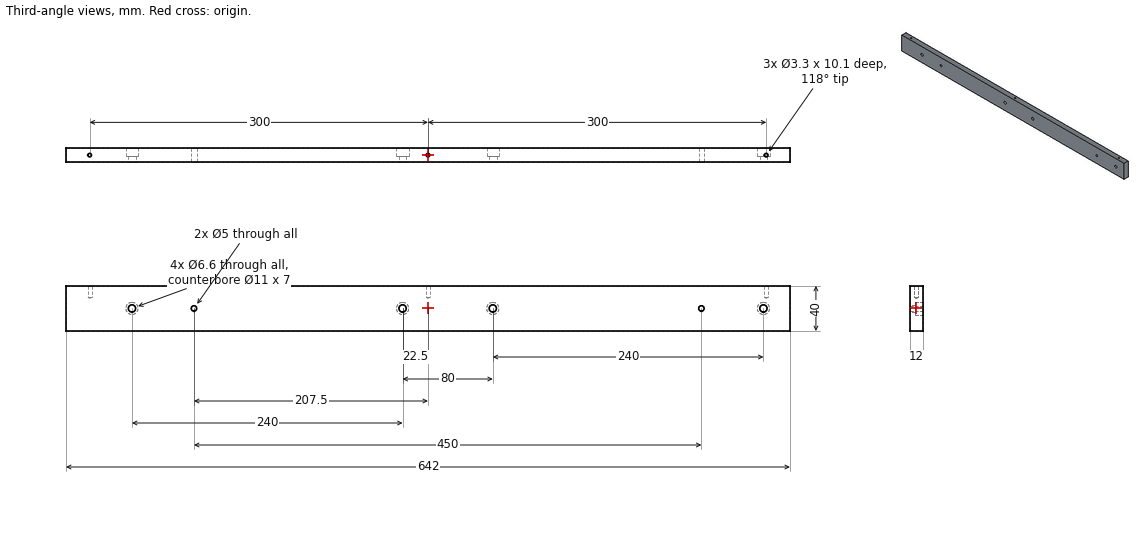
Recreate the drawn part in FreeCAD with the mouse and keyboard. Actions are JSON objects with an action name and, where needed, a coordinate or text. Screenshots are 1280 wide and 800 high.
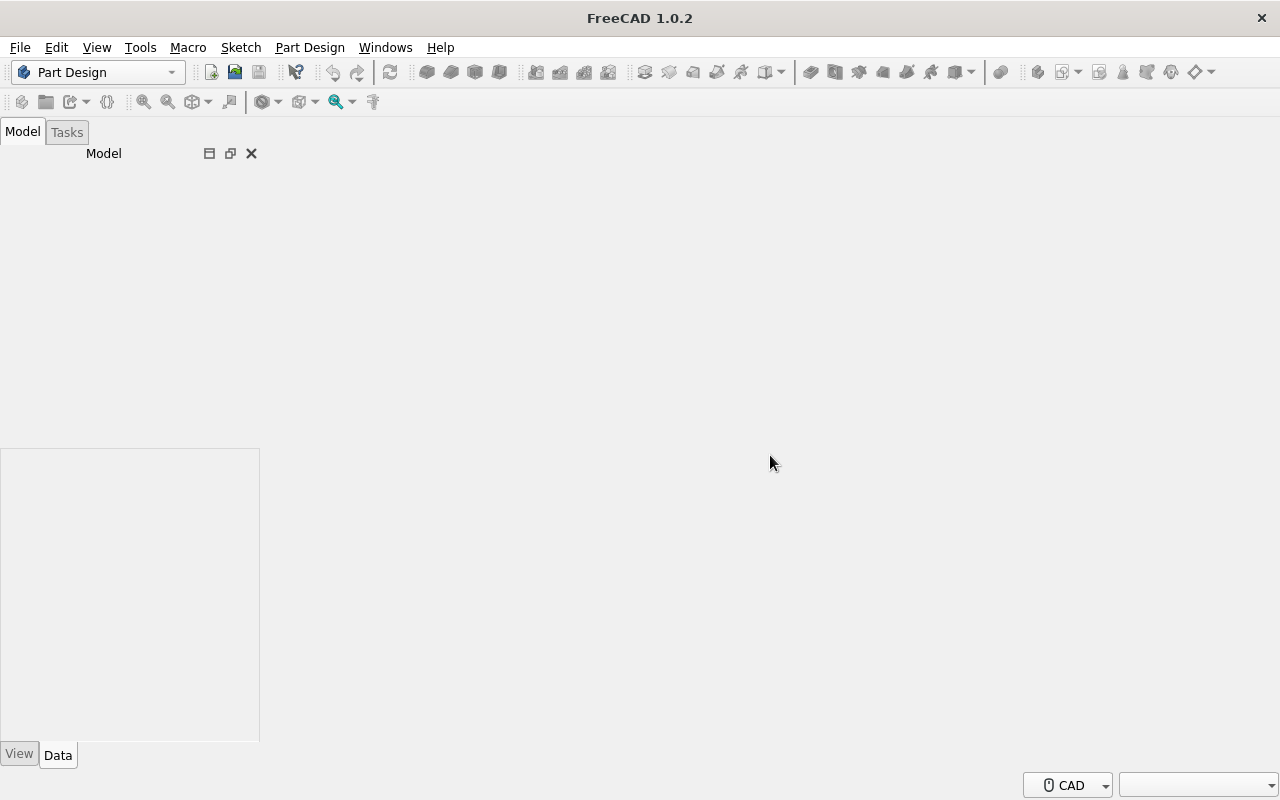
{"action": "left_click", "coordinate": [212, 72]}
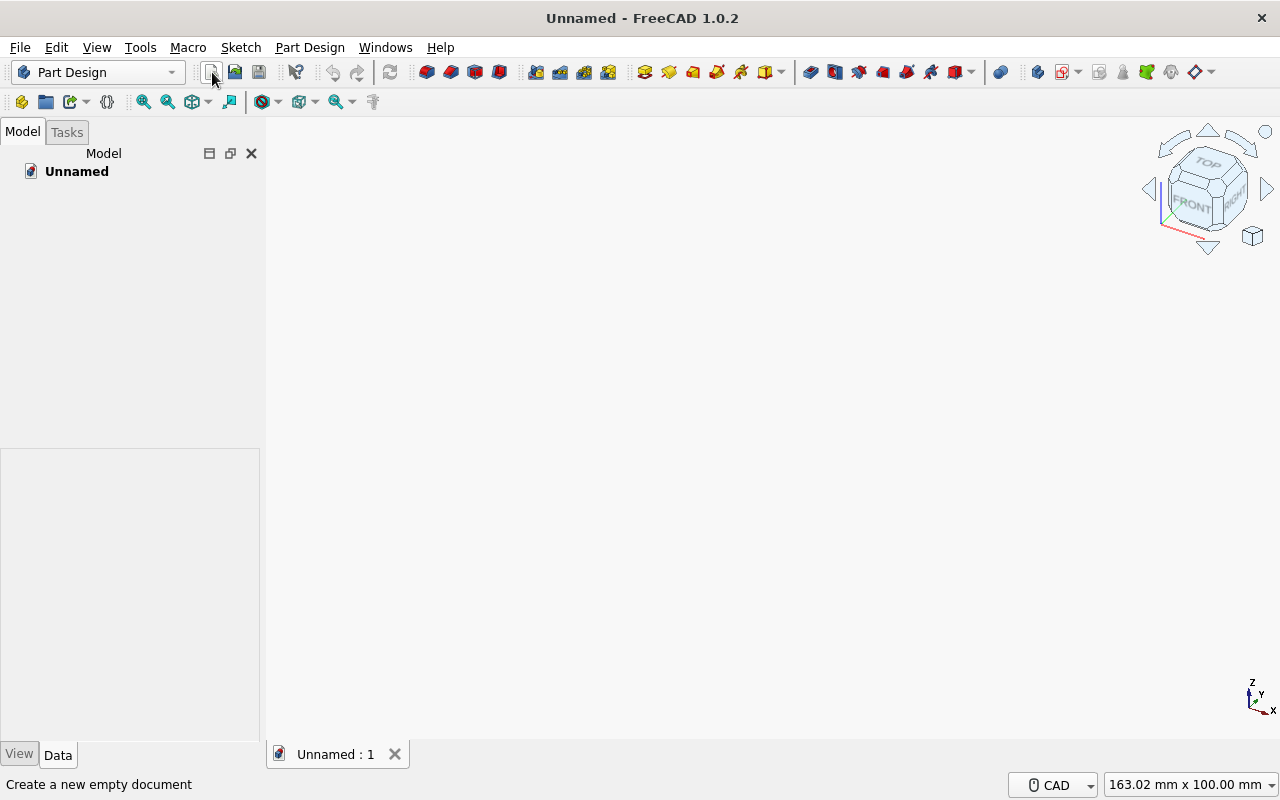
{"action": "left_click", "coordinate": [1062, 72]}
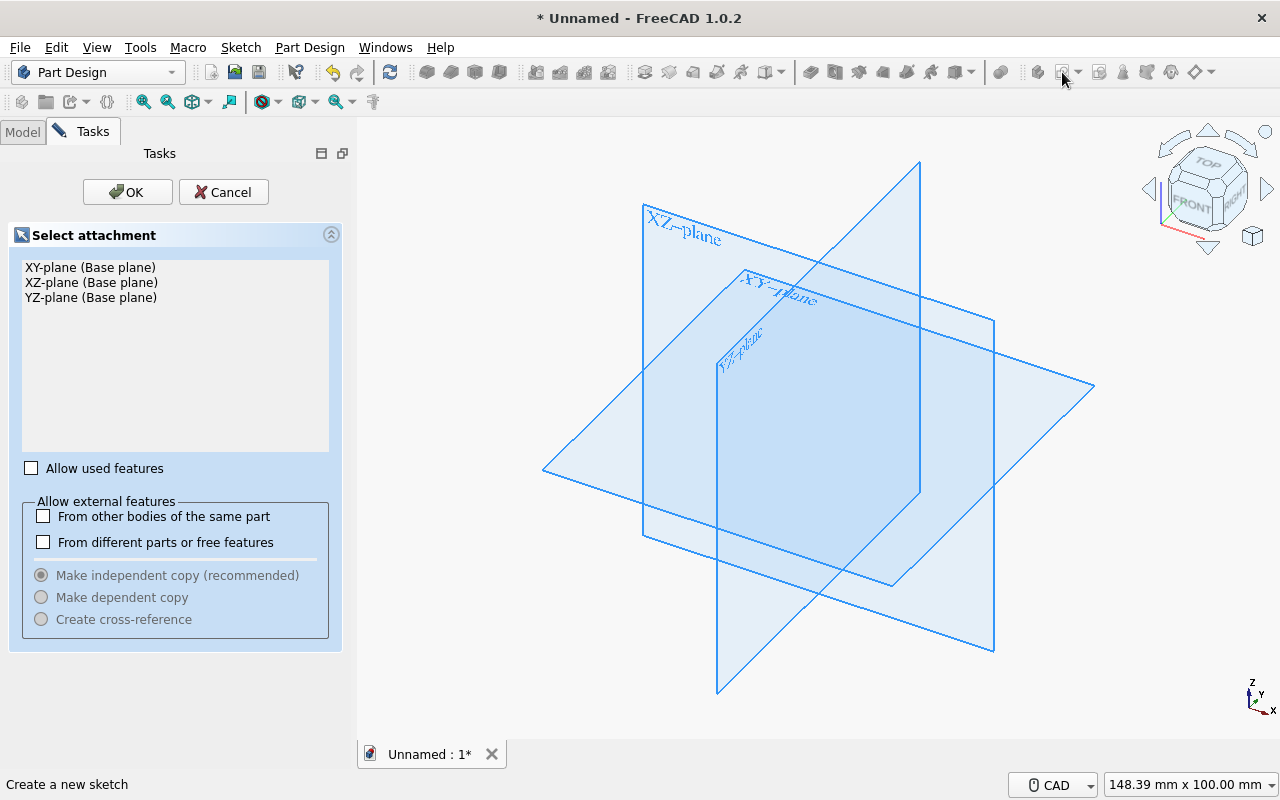
{"action": "left_click", "coordinate": [82, 282]}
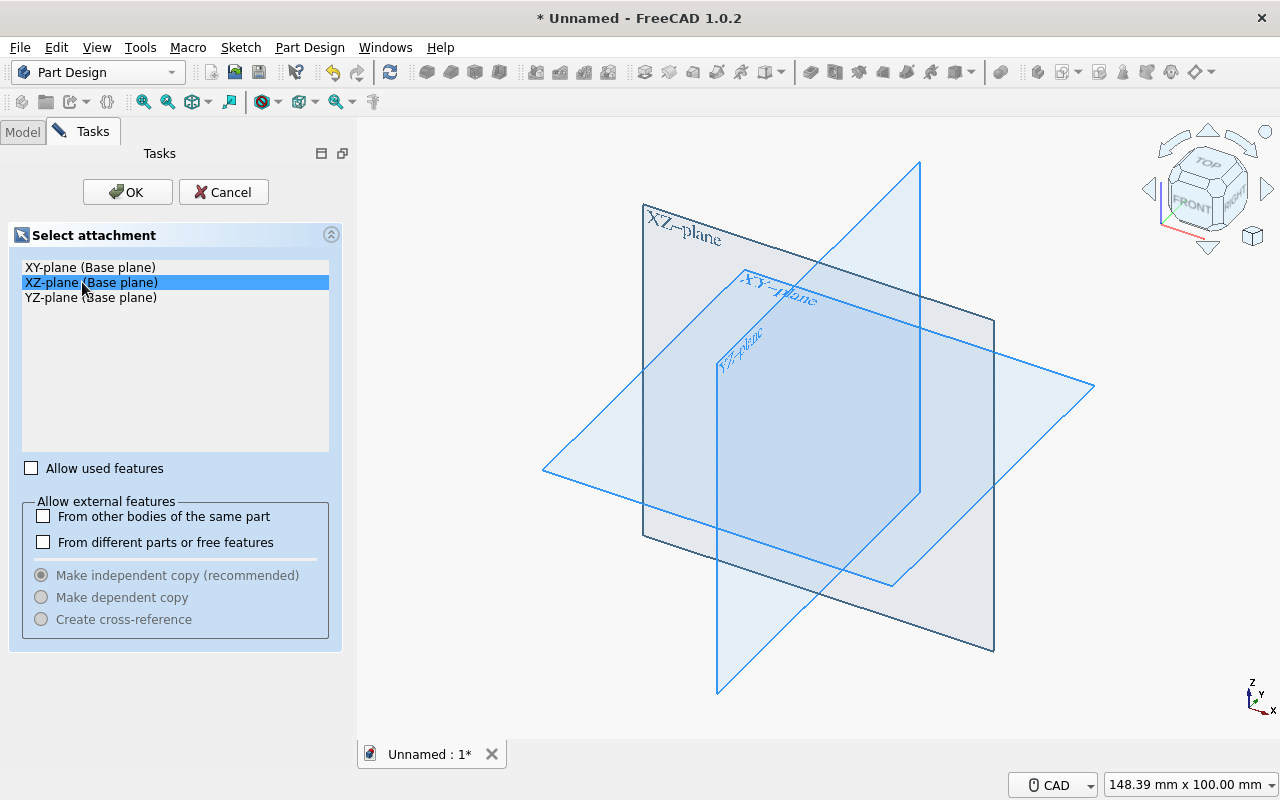
{"action": "left_click", "coordinate": [128, 192]}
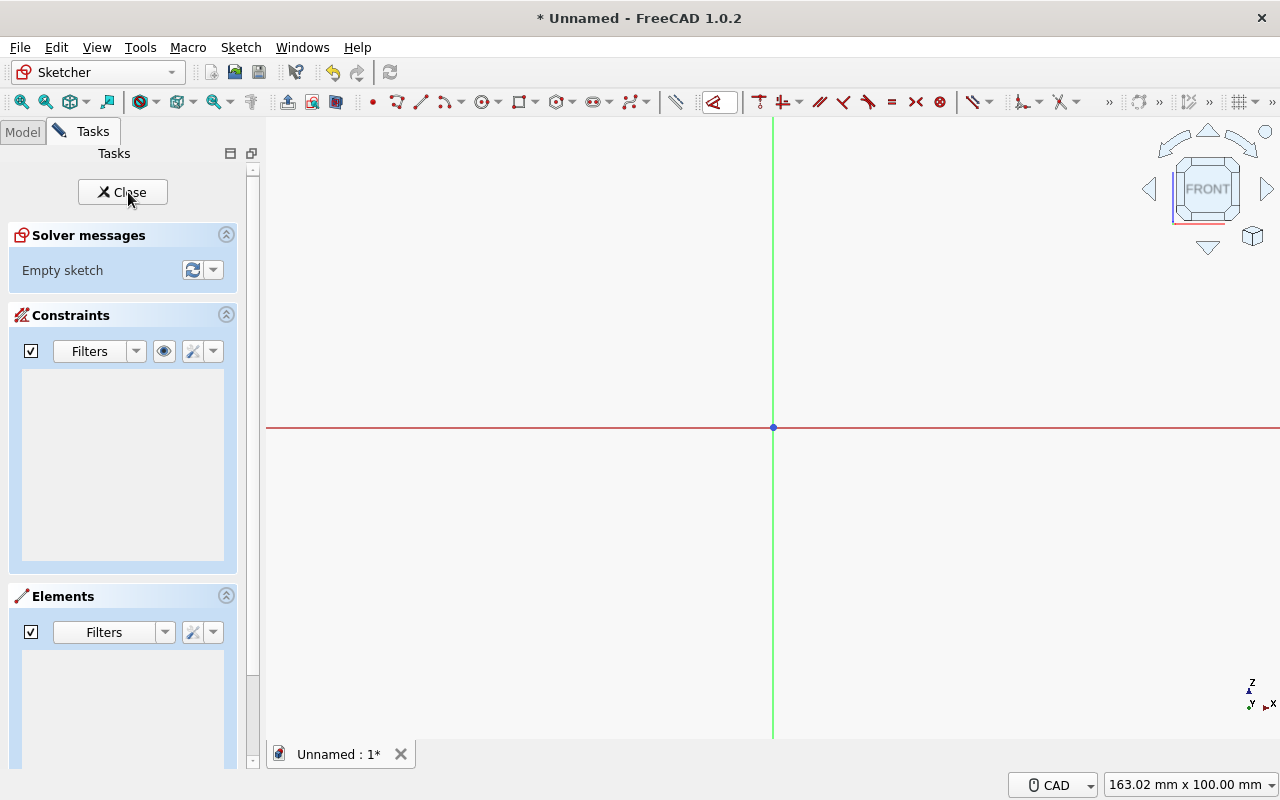
{"action": "scroll", "coordinate": [694, 428], "scroll_direction": "down", "scroll_amount": 10}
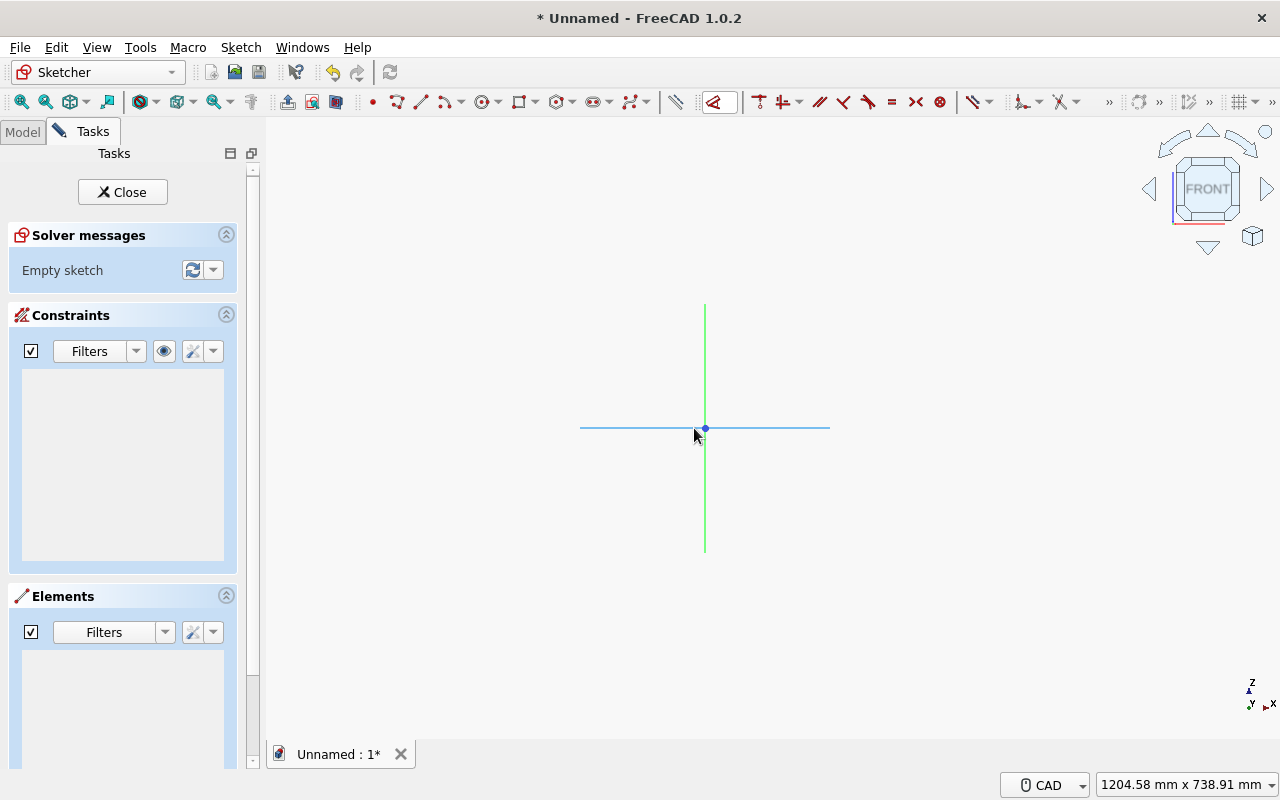
{"action": "left_click", "coordinate": [538, 102]}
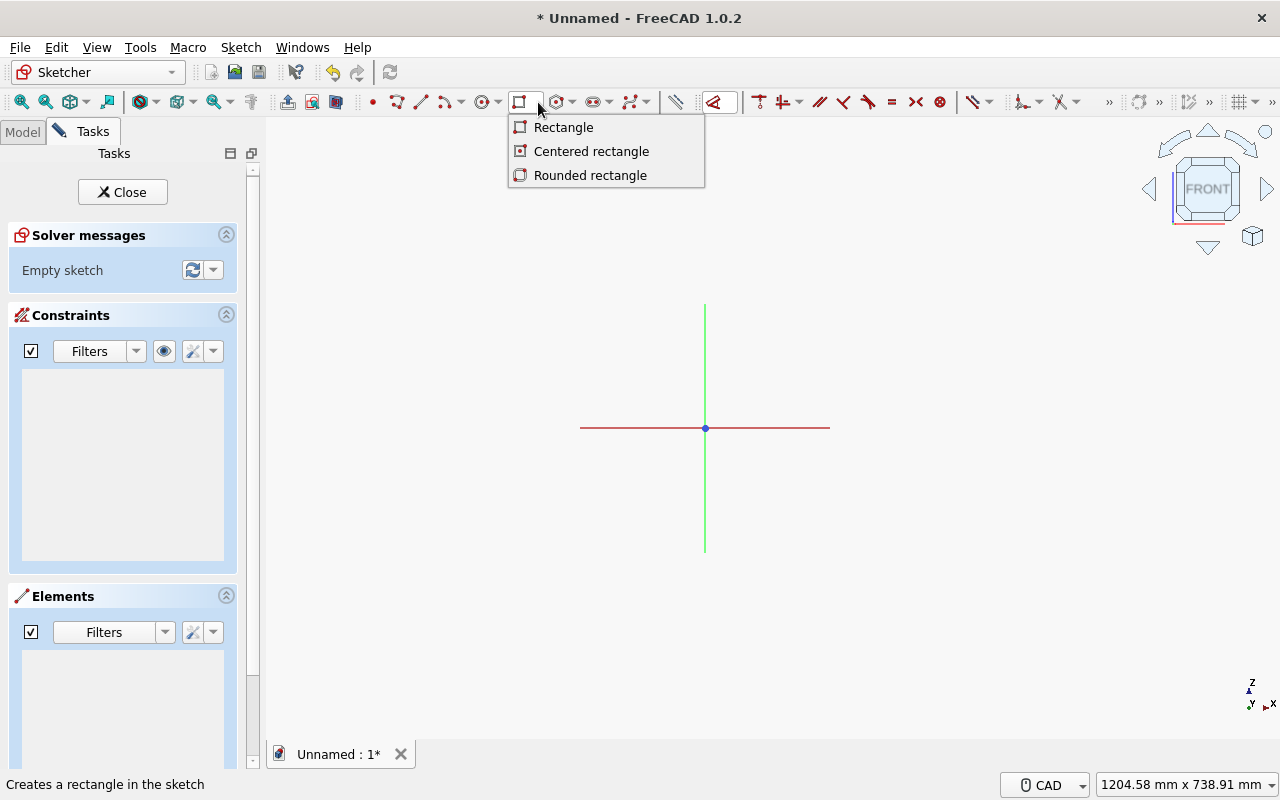
{"action": "left_click", "coordinate": [606, 151]}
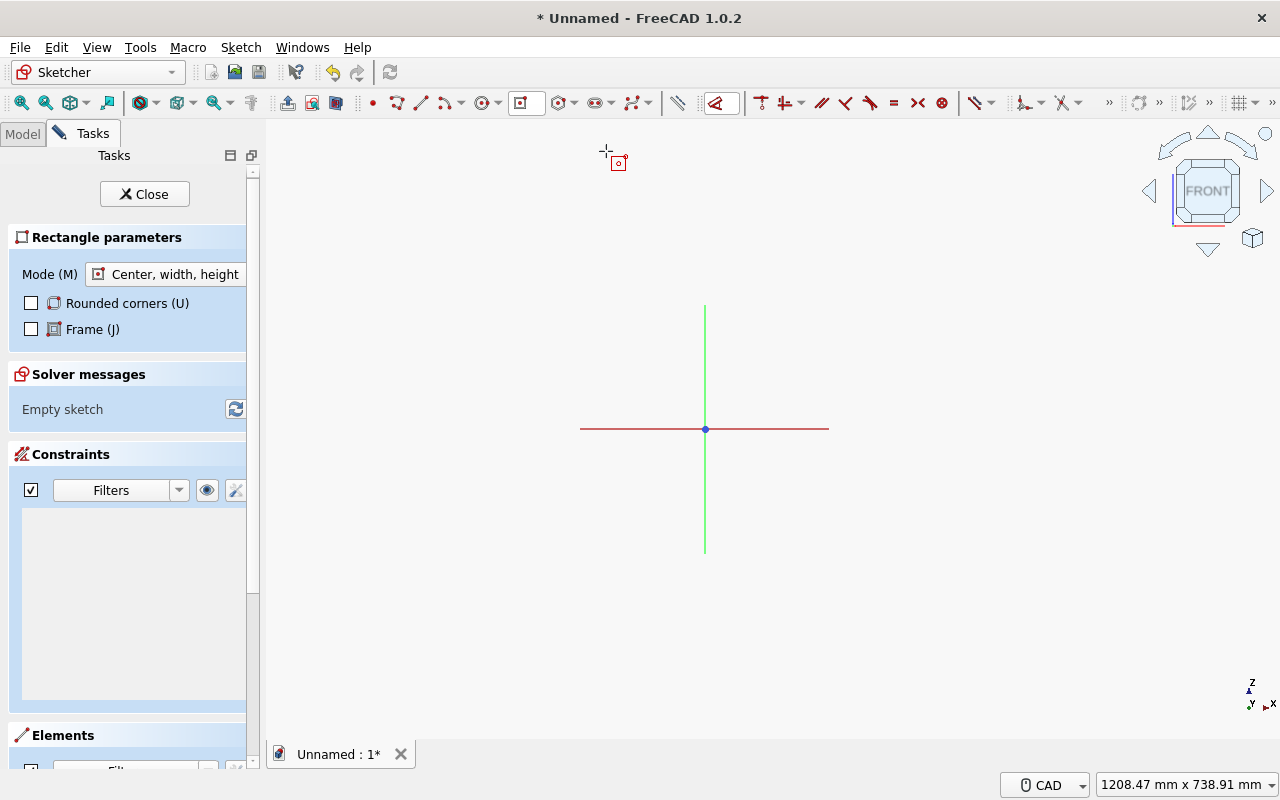
{"action": "left_click", "coordinate": [705, 429]}
{"action": "left_click", "coordinate": [975, 413]}
{"action": "key", "text": "Escape"}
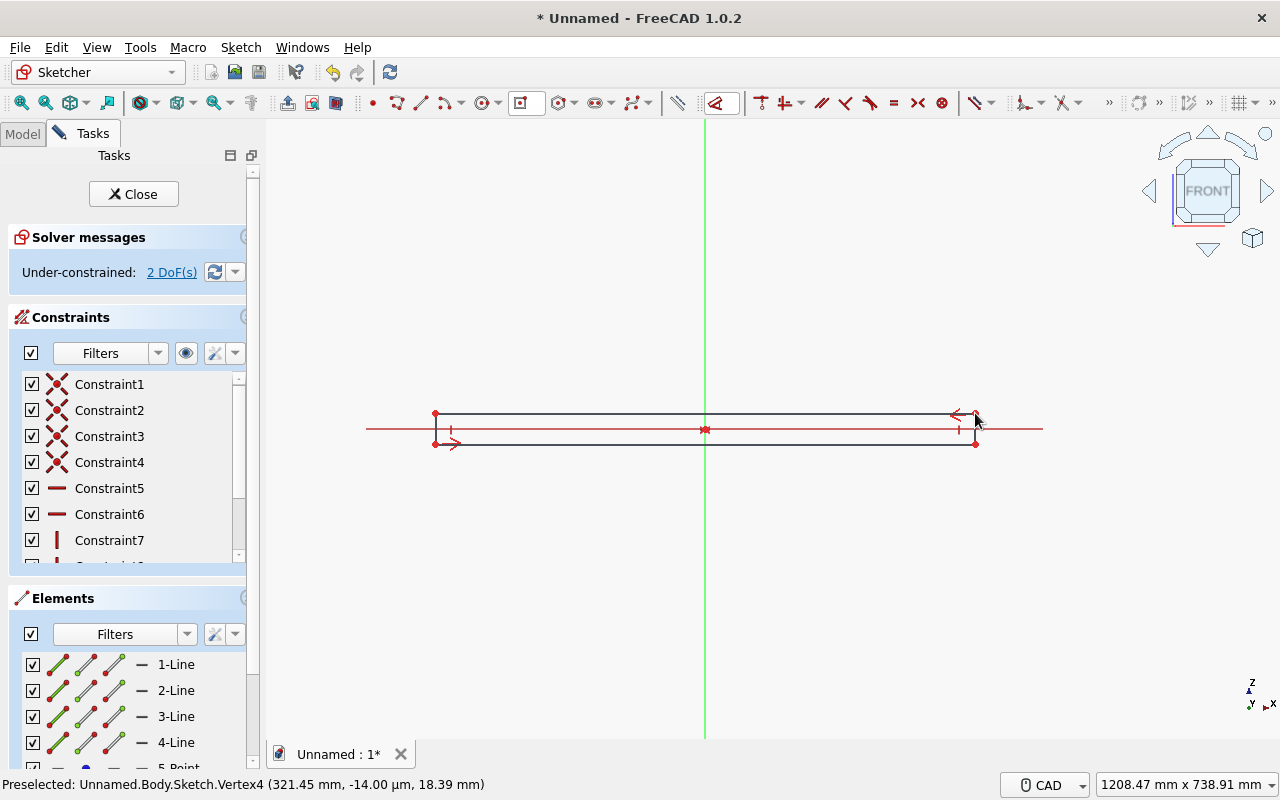
{"action": "left_click", "coordinate": [716, 104]}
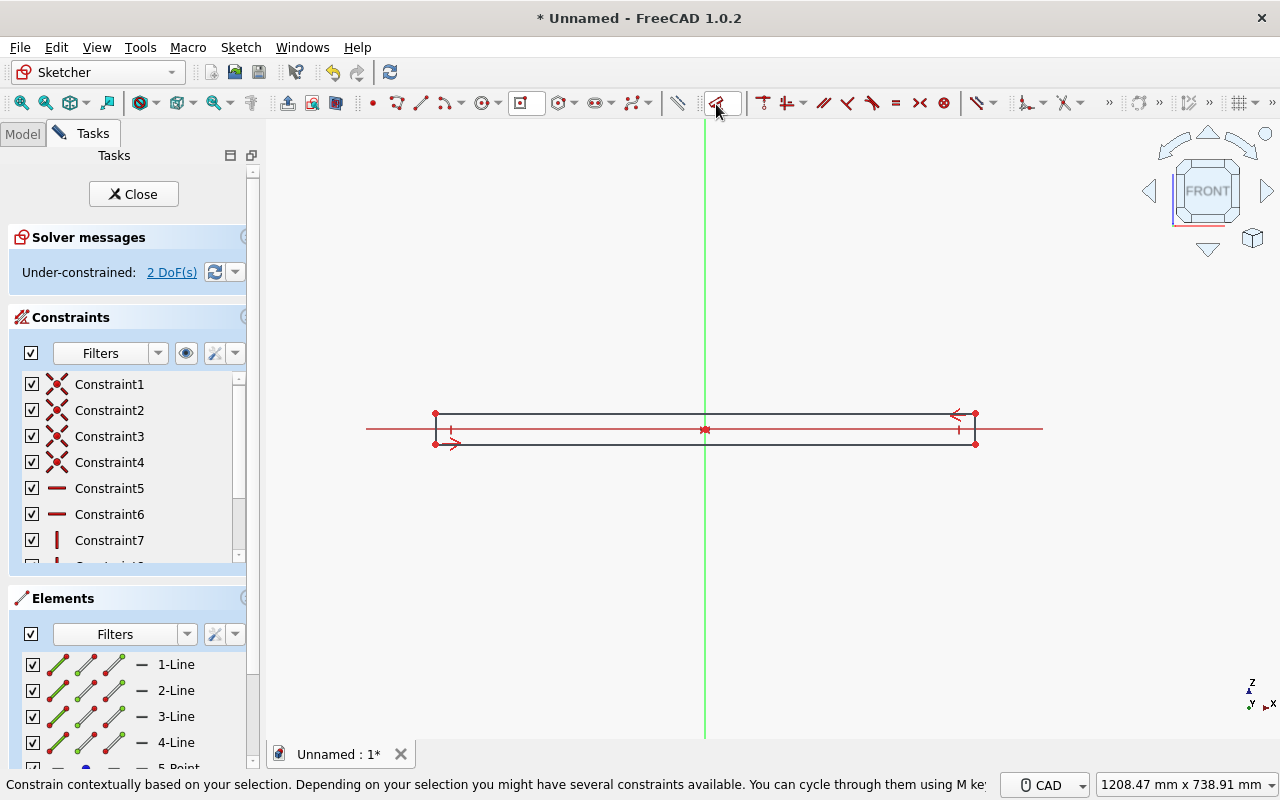
{"action": "left_click", "coordinate": [975, 433]}
{"action": "left_click", "coordinate": [1009, 422]}